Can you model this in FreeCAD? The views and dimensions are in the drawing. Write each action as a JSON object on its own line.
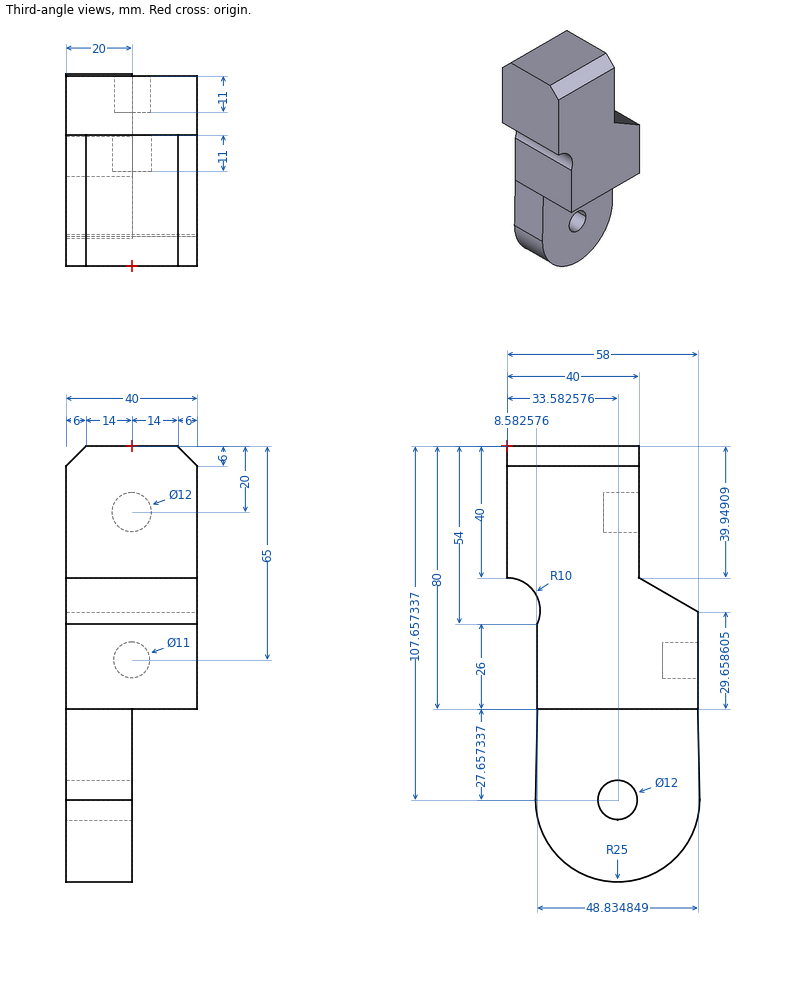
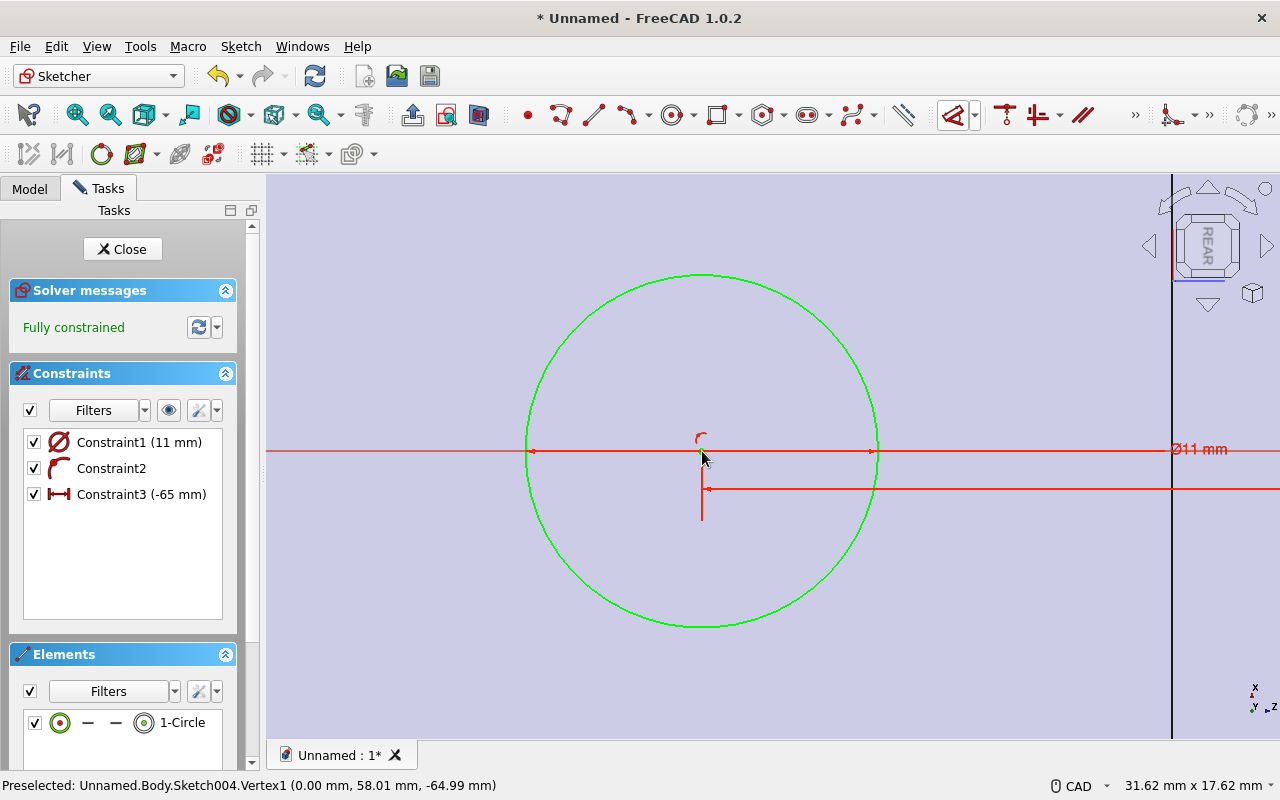
{"action": "left_click", "coordinate": [123, 249]}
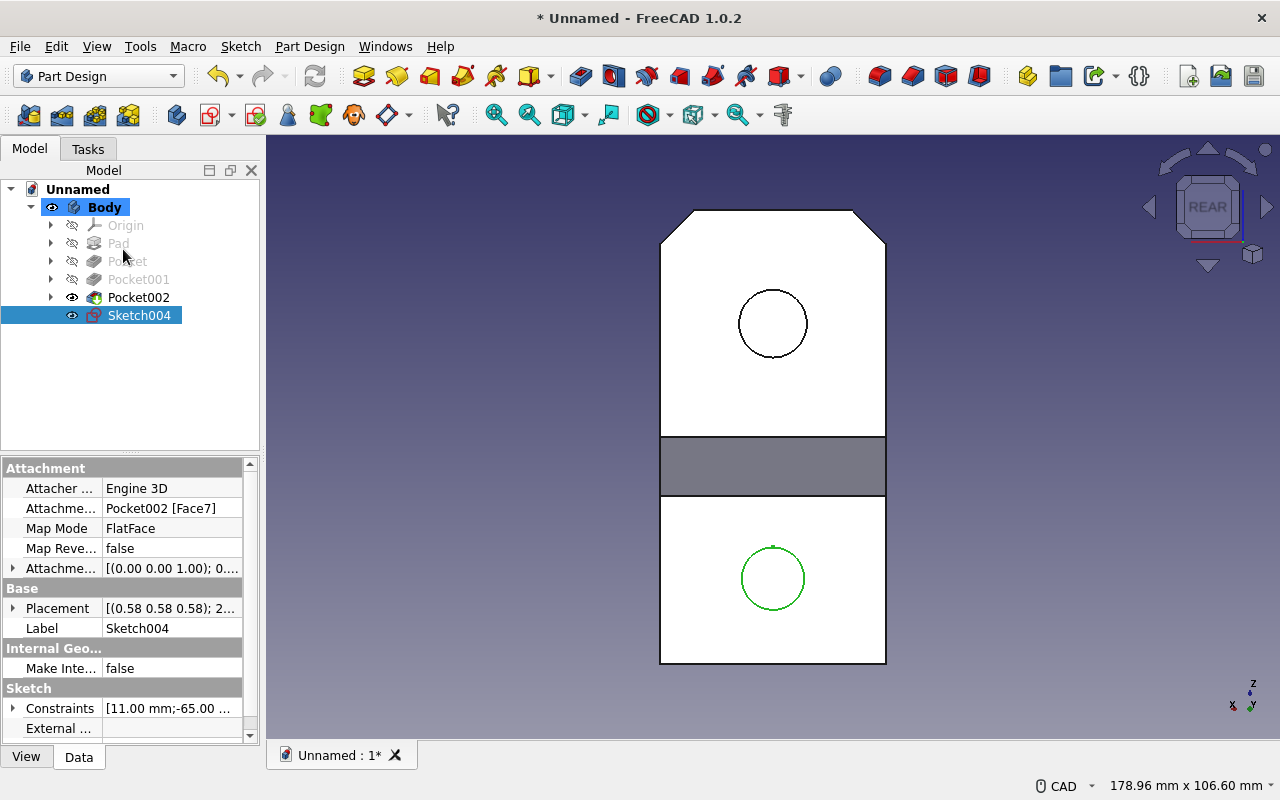
{"action": "left_click", "coordinate": [581, 76]}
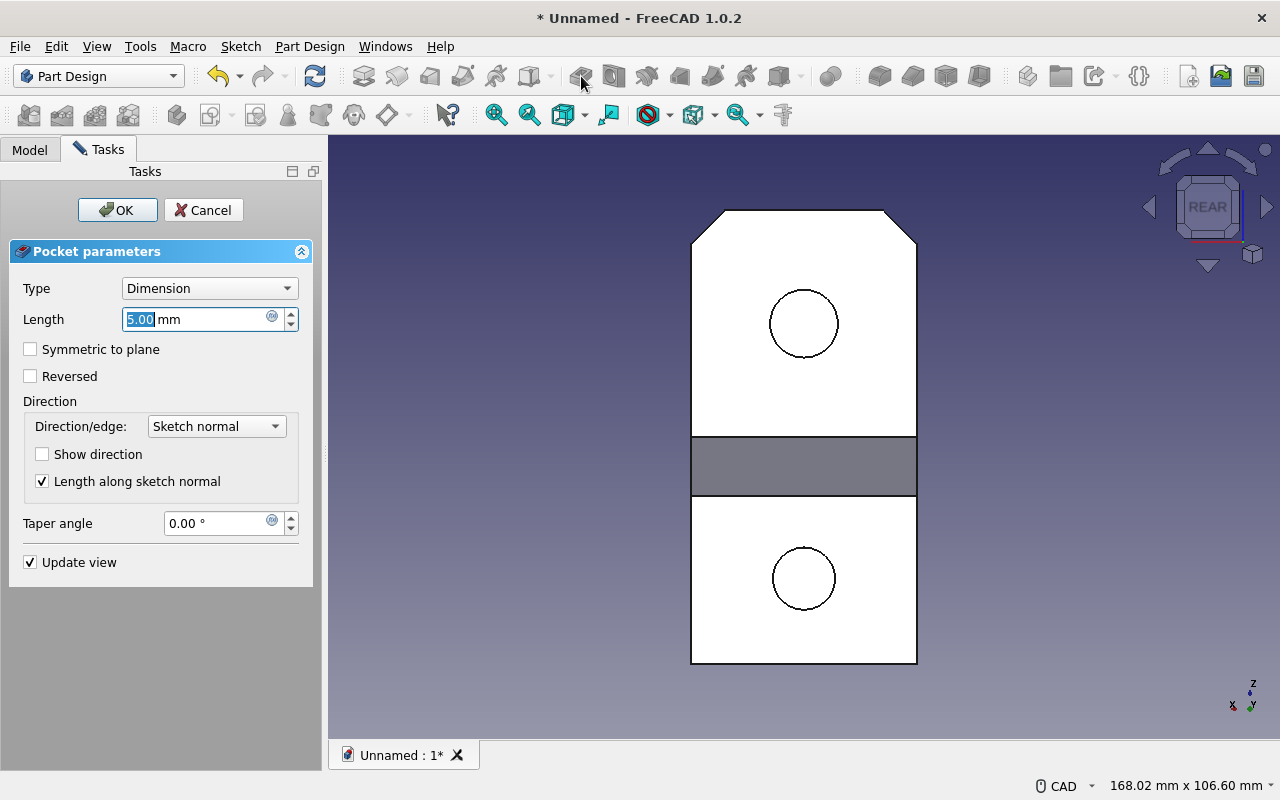
{"action": "type", "text": "11"}
{"action": "key", "text": "Tab"}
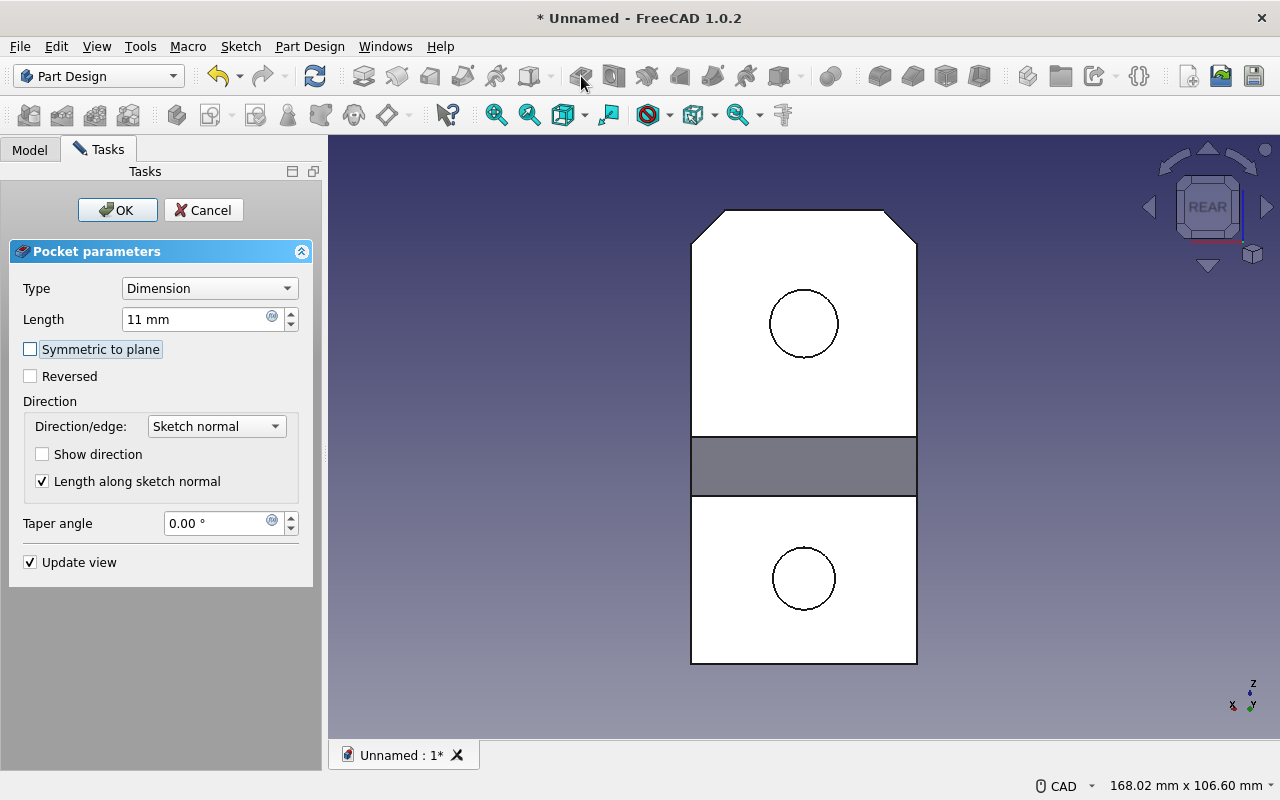
{"action": "left_click", "coordinate": [118, 210]}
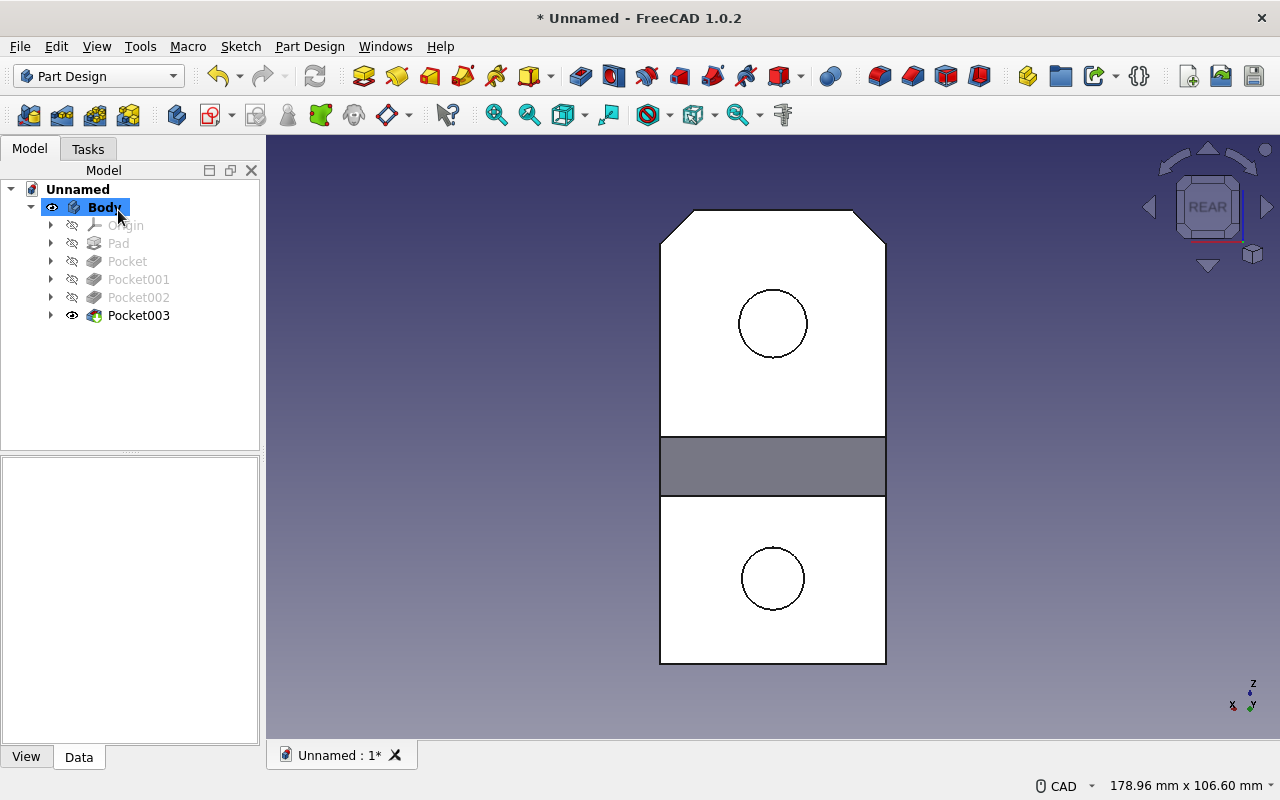
{"action": "key", "text": "6"}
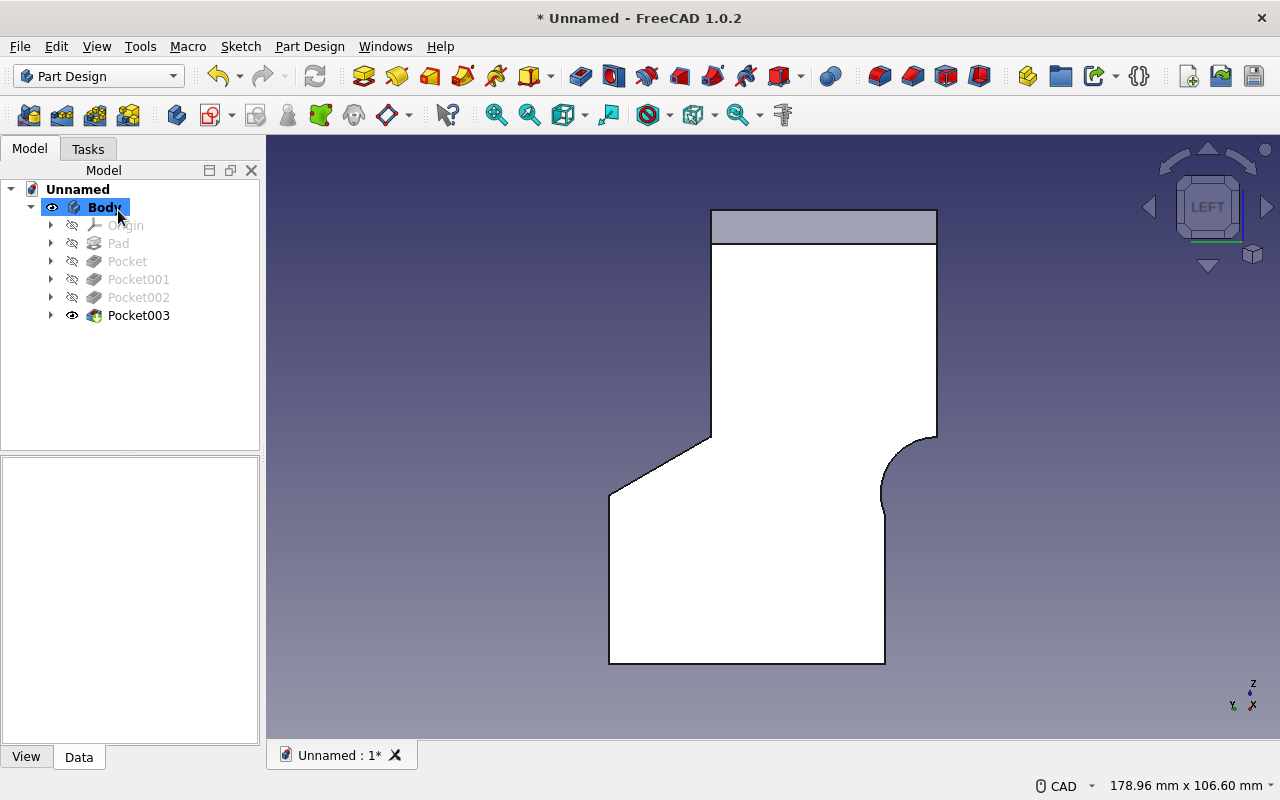
{"action": "left_click", "coordinate": [773, 513]}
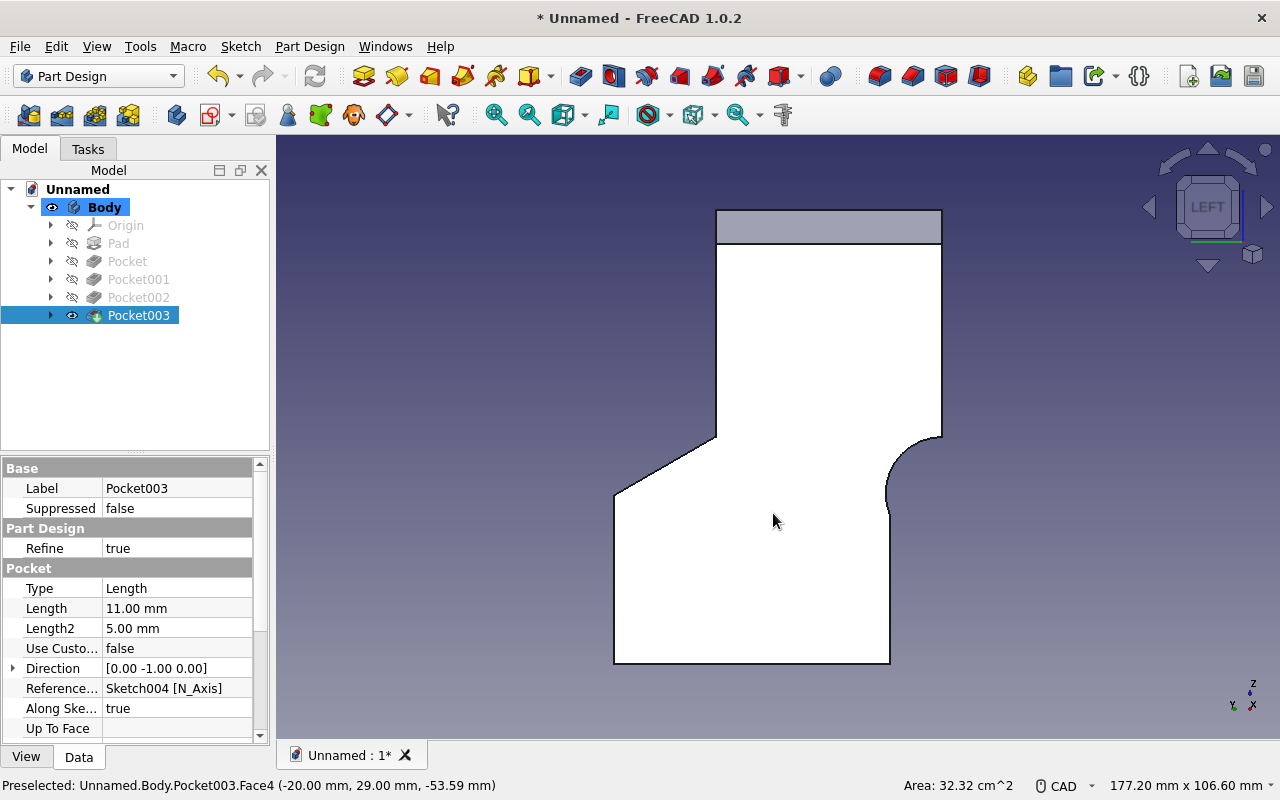
{"action": "left_click", "coordinate": [210, 116]}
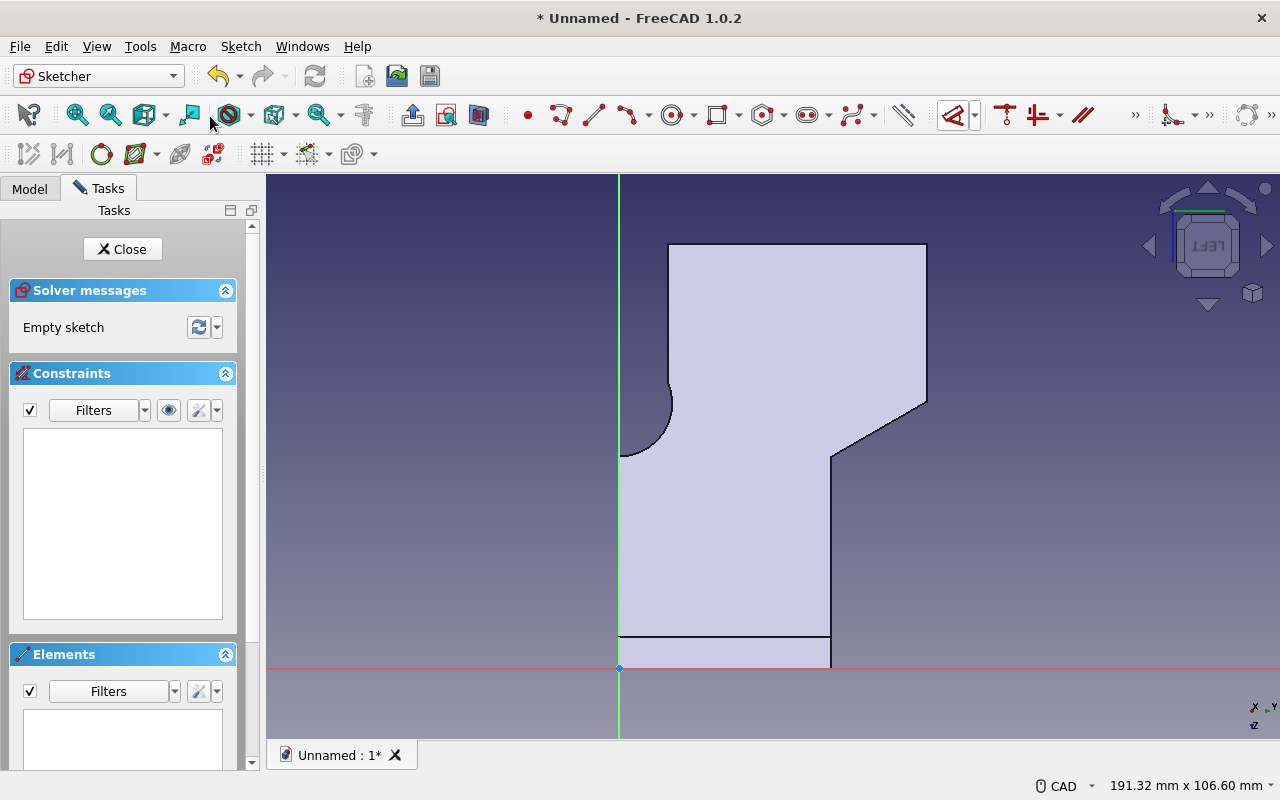
{"action": "scroll", "coordinate": [704, 456], "scroll_direction": "down", "scroll_amount": 5}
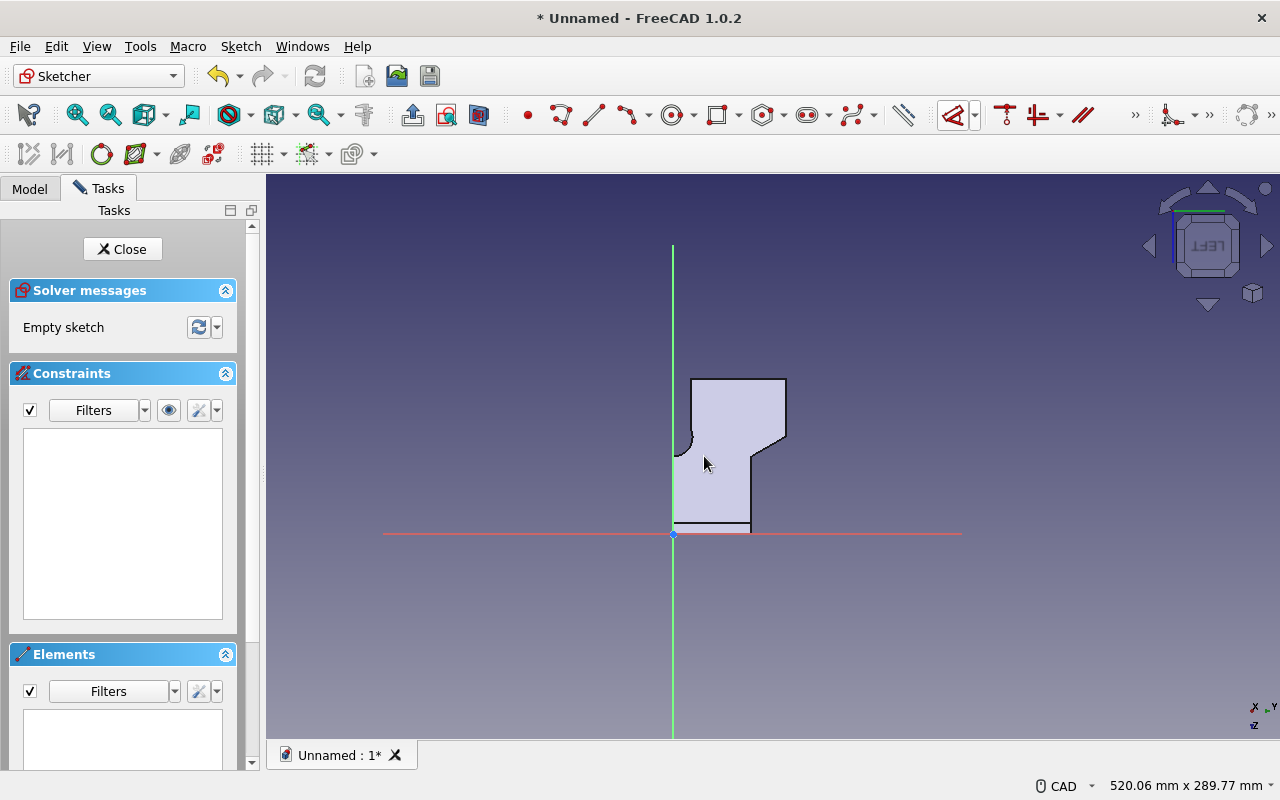
{"action": "scroll", "coordinate": [753, 271], "scroll_direction": "up", "scroll_amount": 6}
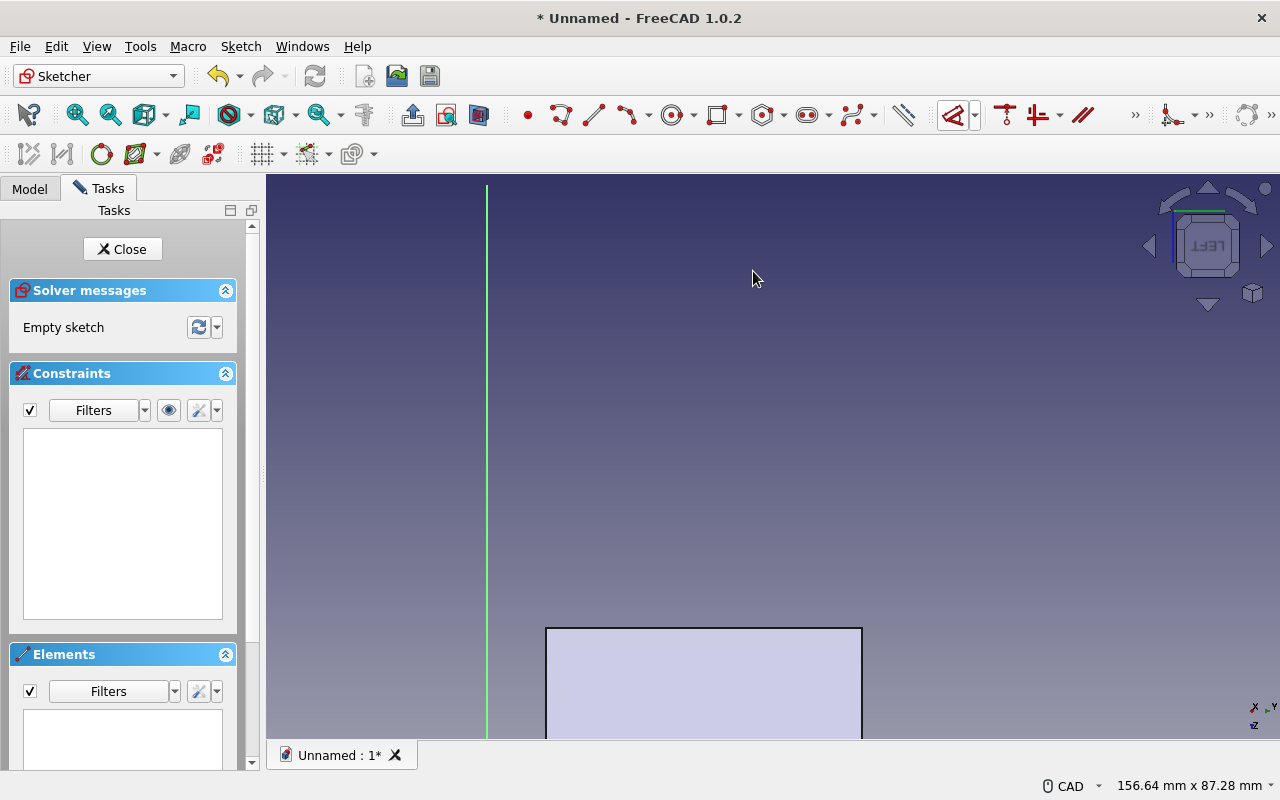
{"action": "key", "text": "g m"}